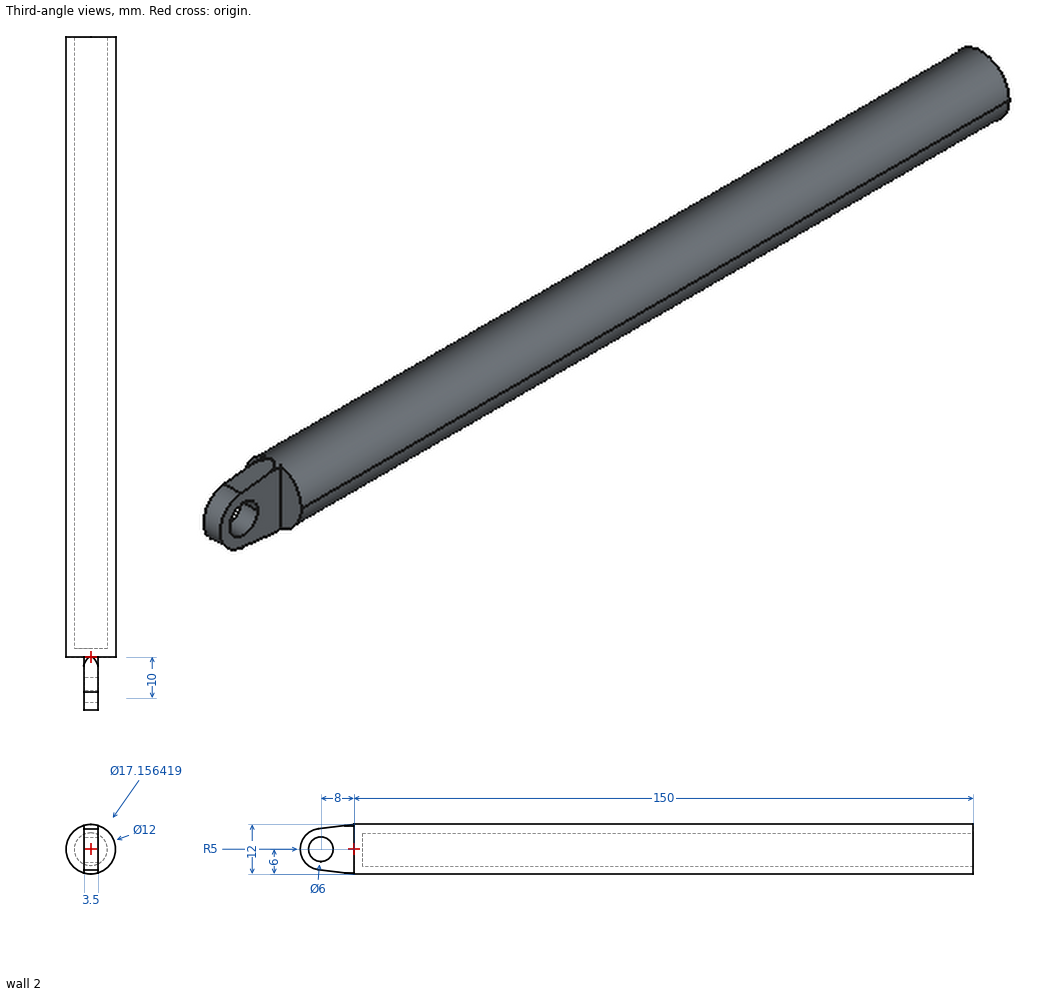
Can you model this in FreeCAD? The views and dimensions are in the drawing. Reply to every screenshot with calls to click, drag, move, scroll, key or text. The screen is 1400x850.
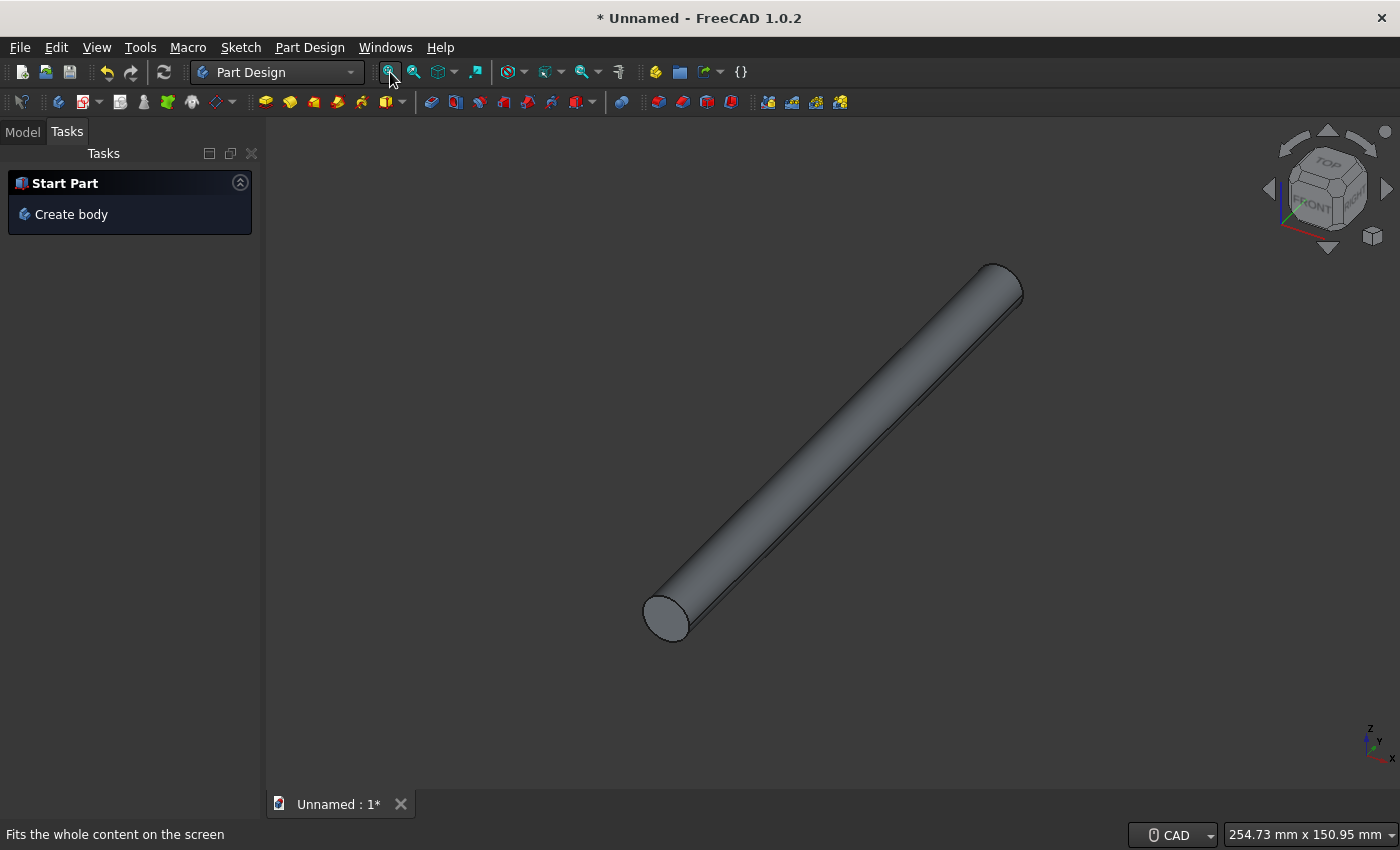
key(0)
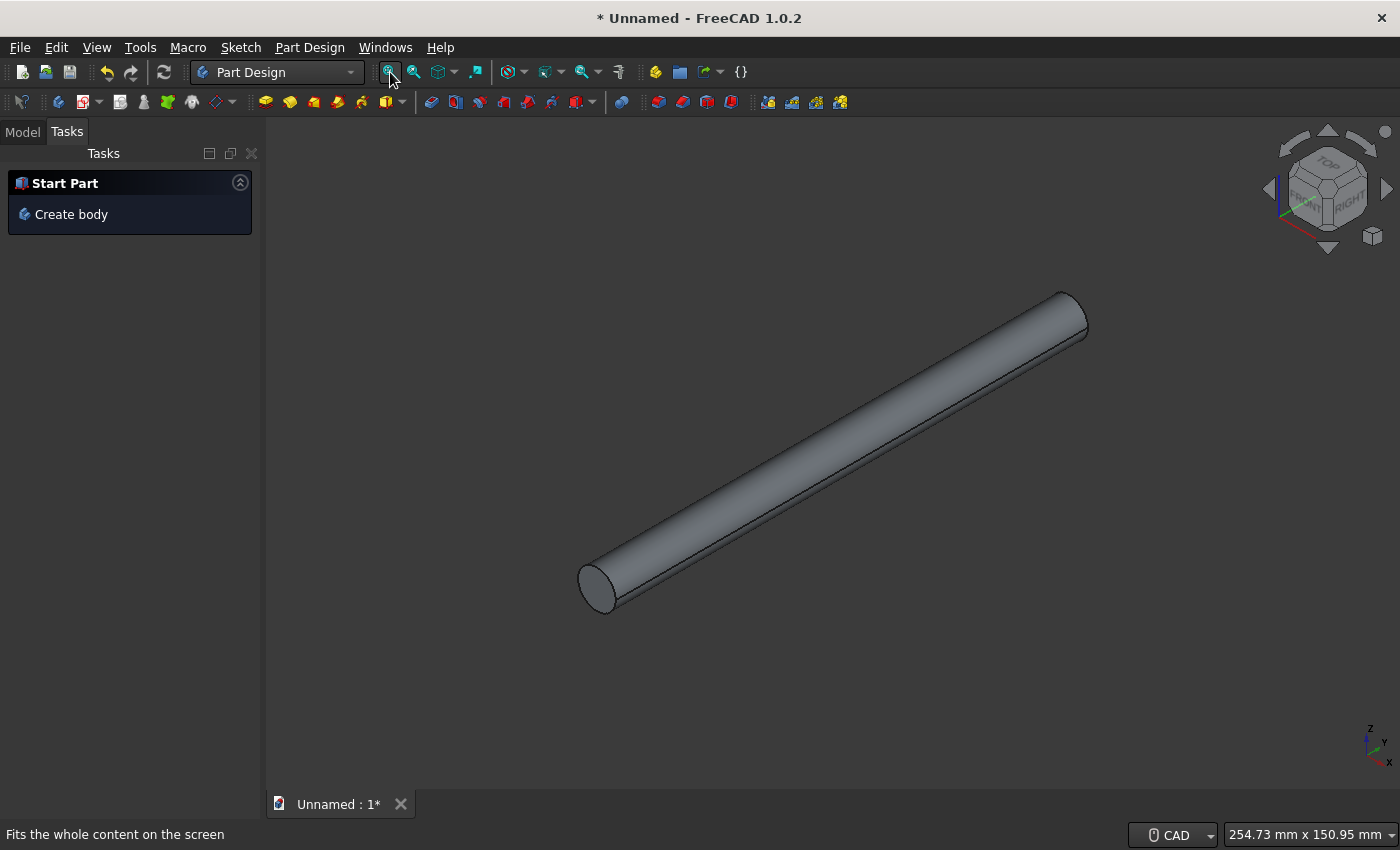
key(2)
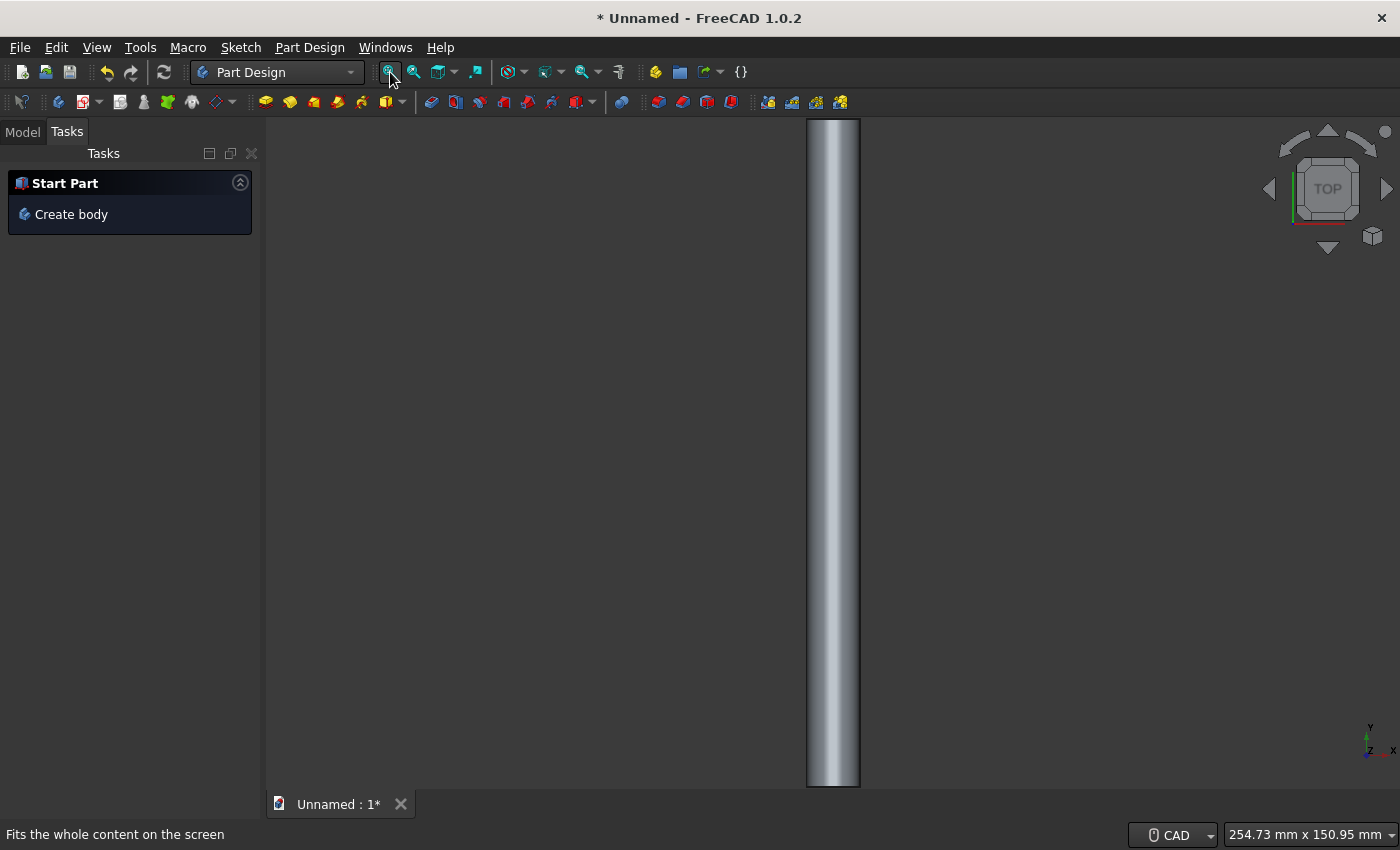
key(1)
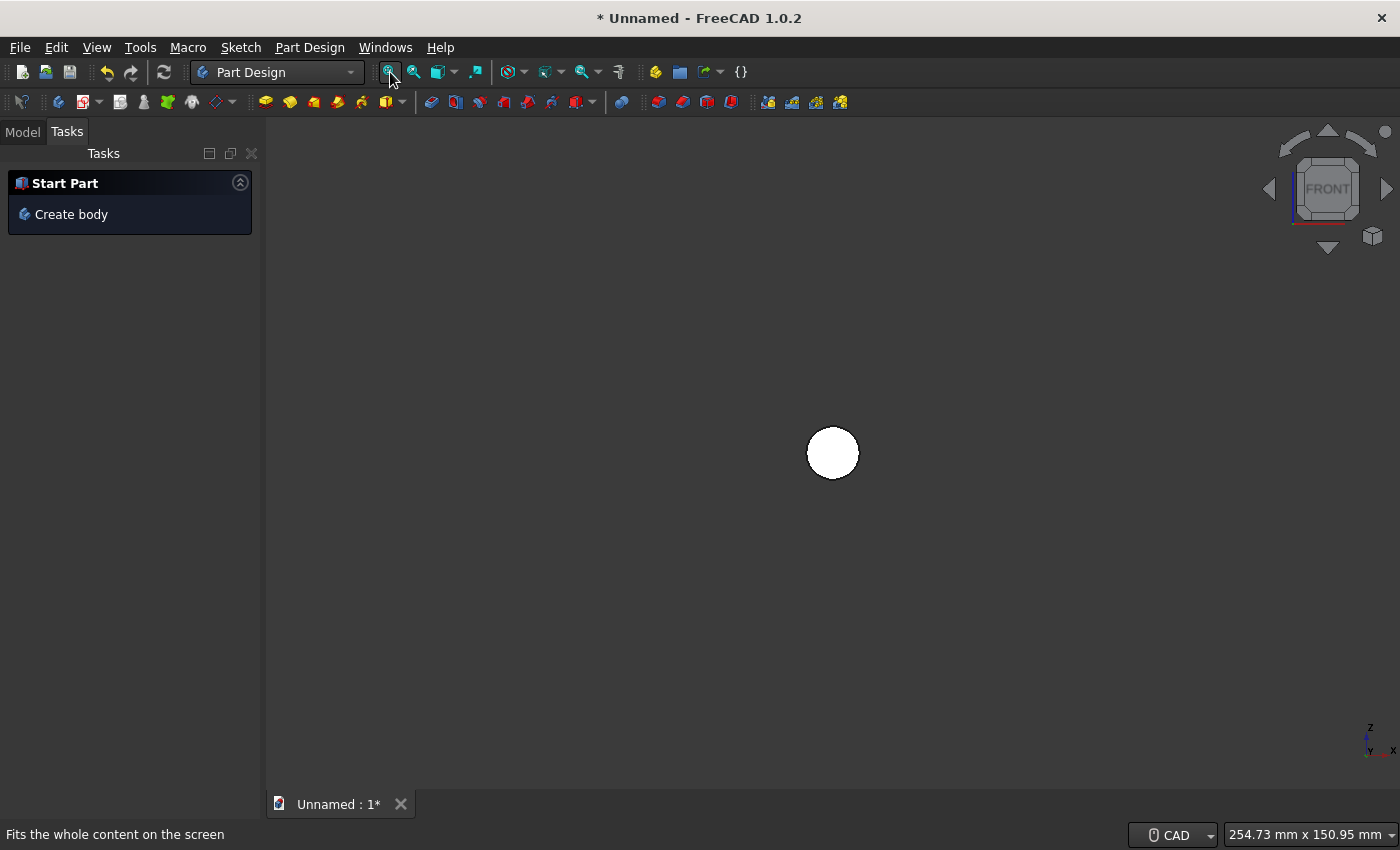
click(390, 72)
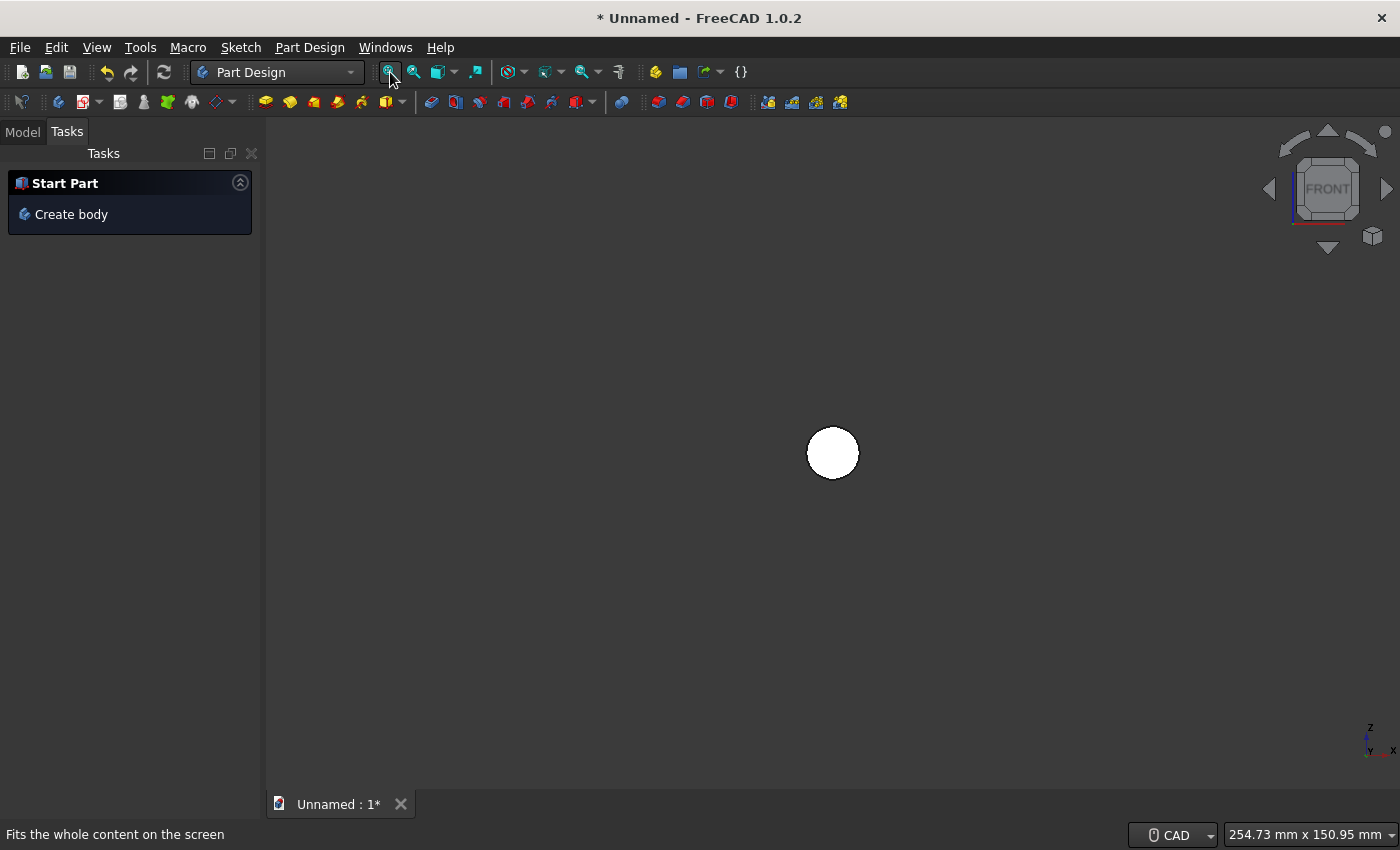
key(3)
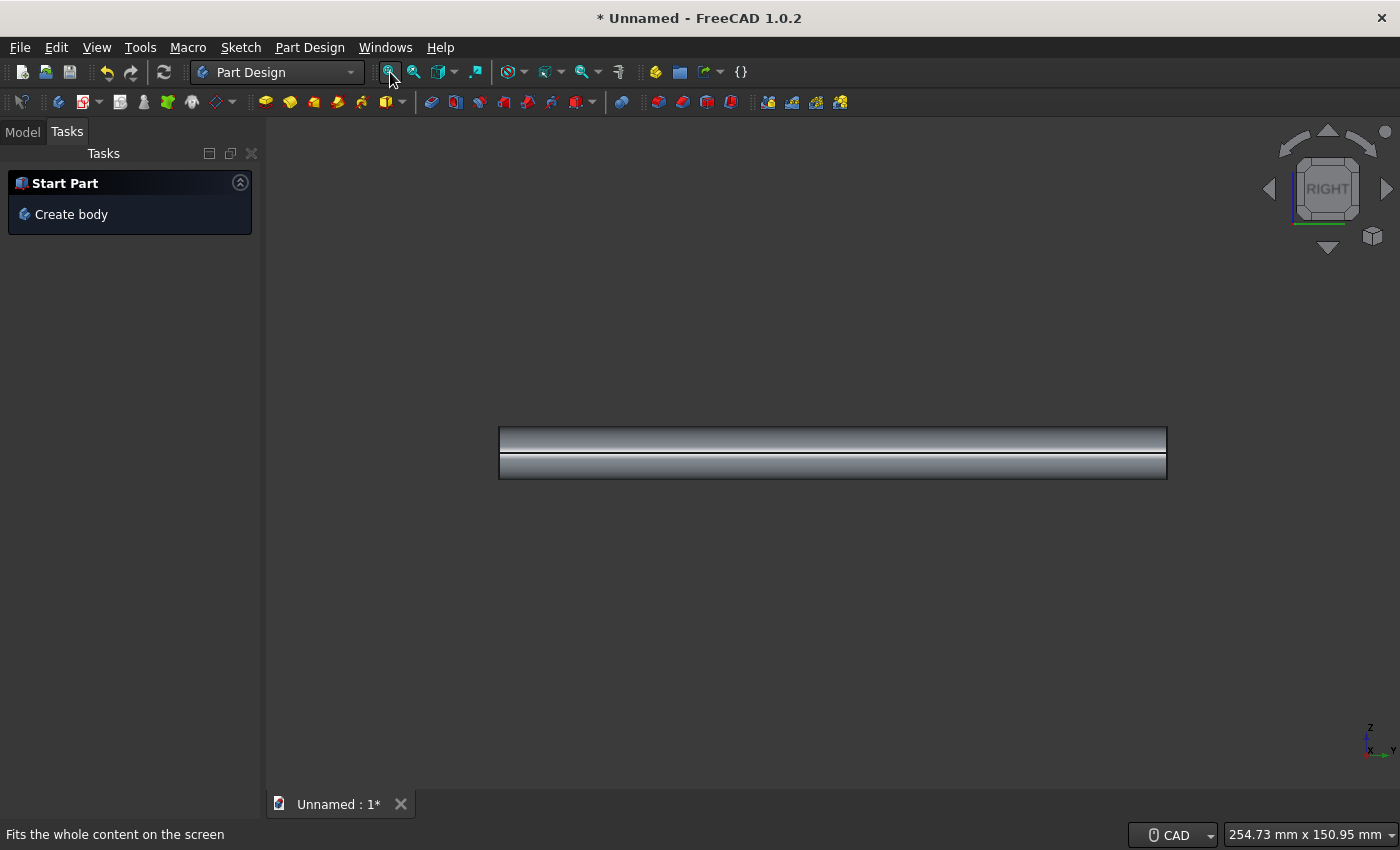
key(5)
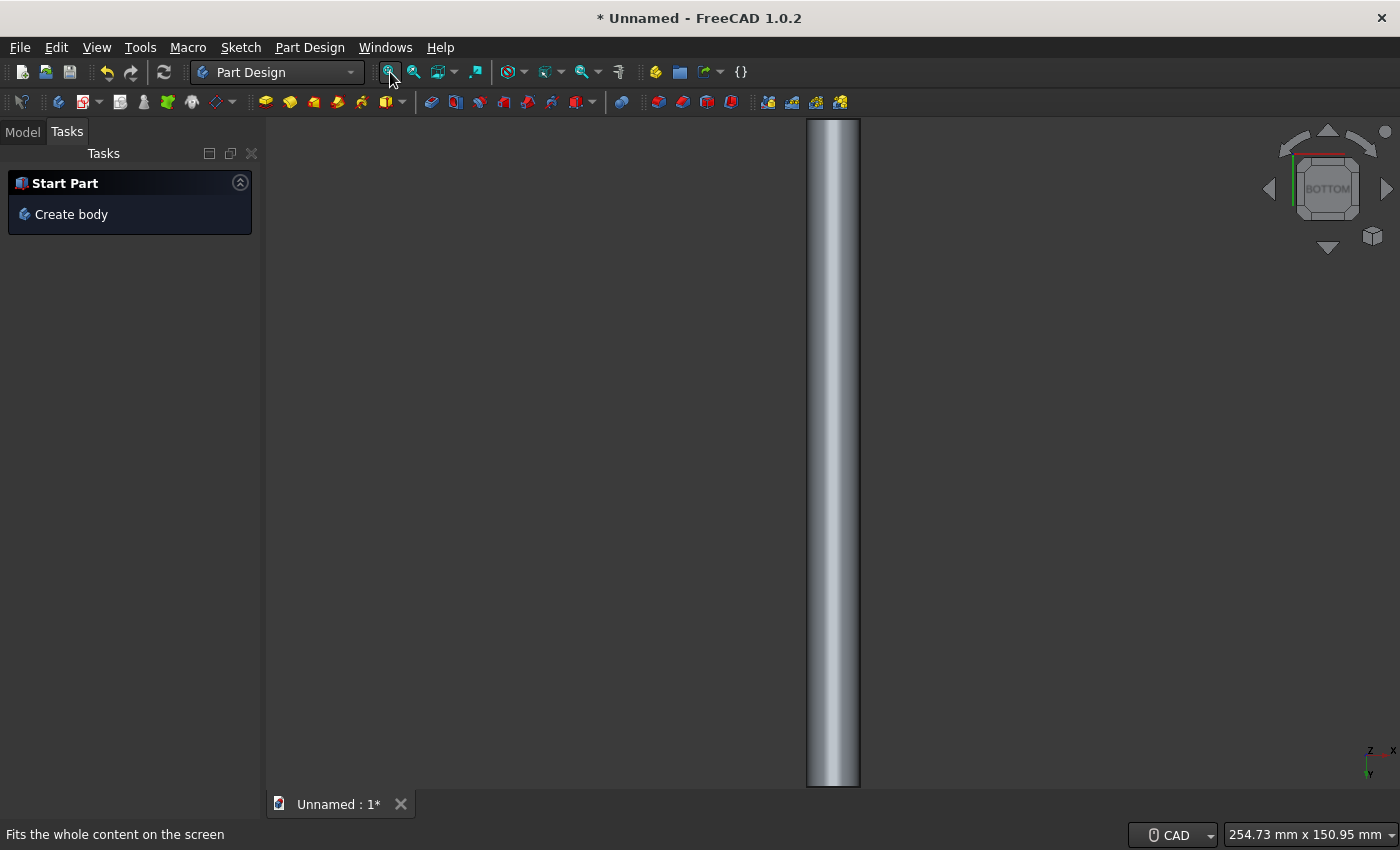
key(4)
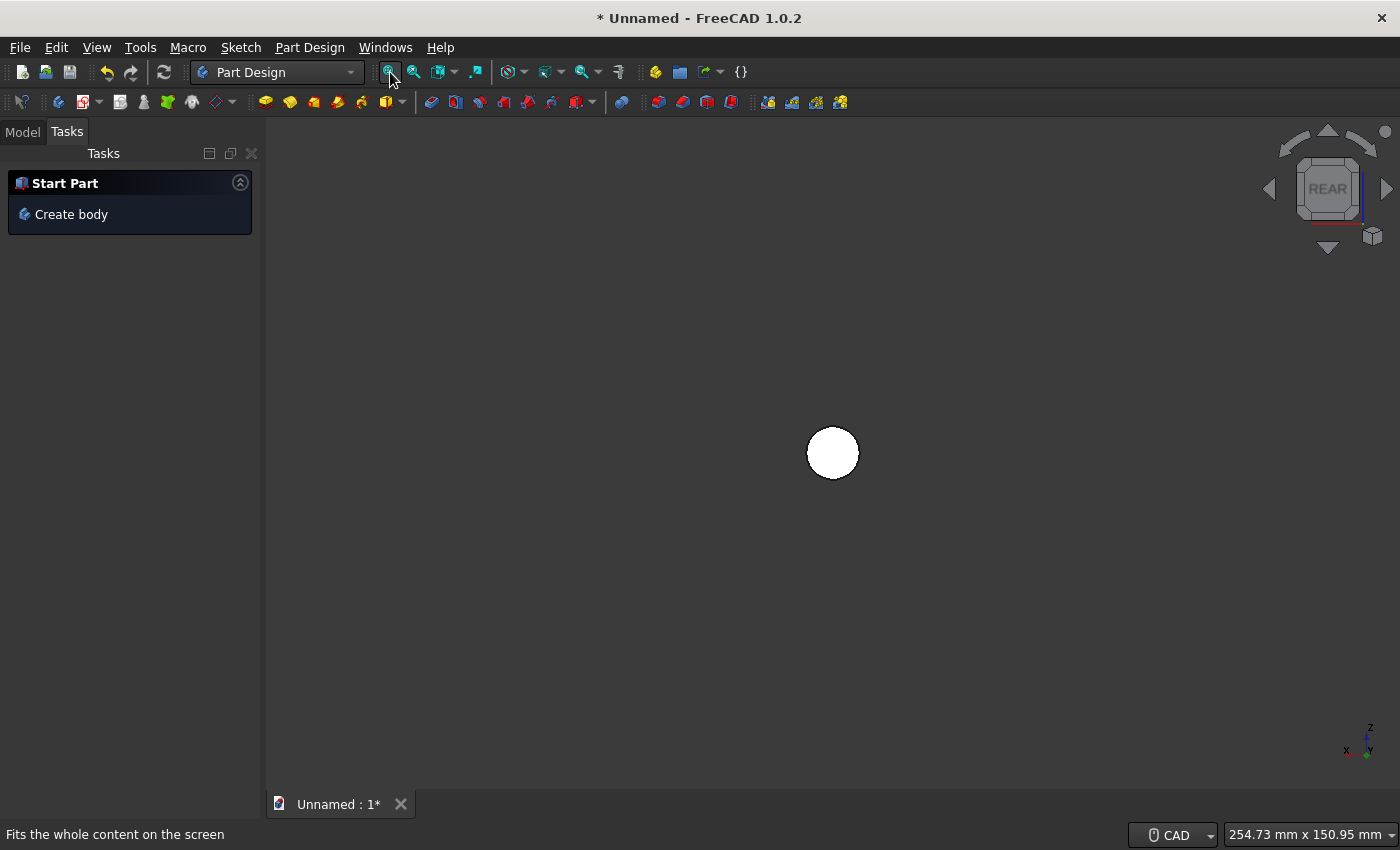
click(390, 72)